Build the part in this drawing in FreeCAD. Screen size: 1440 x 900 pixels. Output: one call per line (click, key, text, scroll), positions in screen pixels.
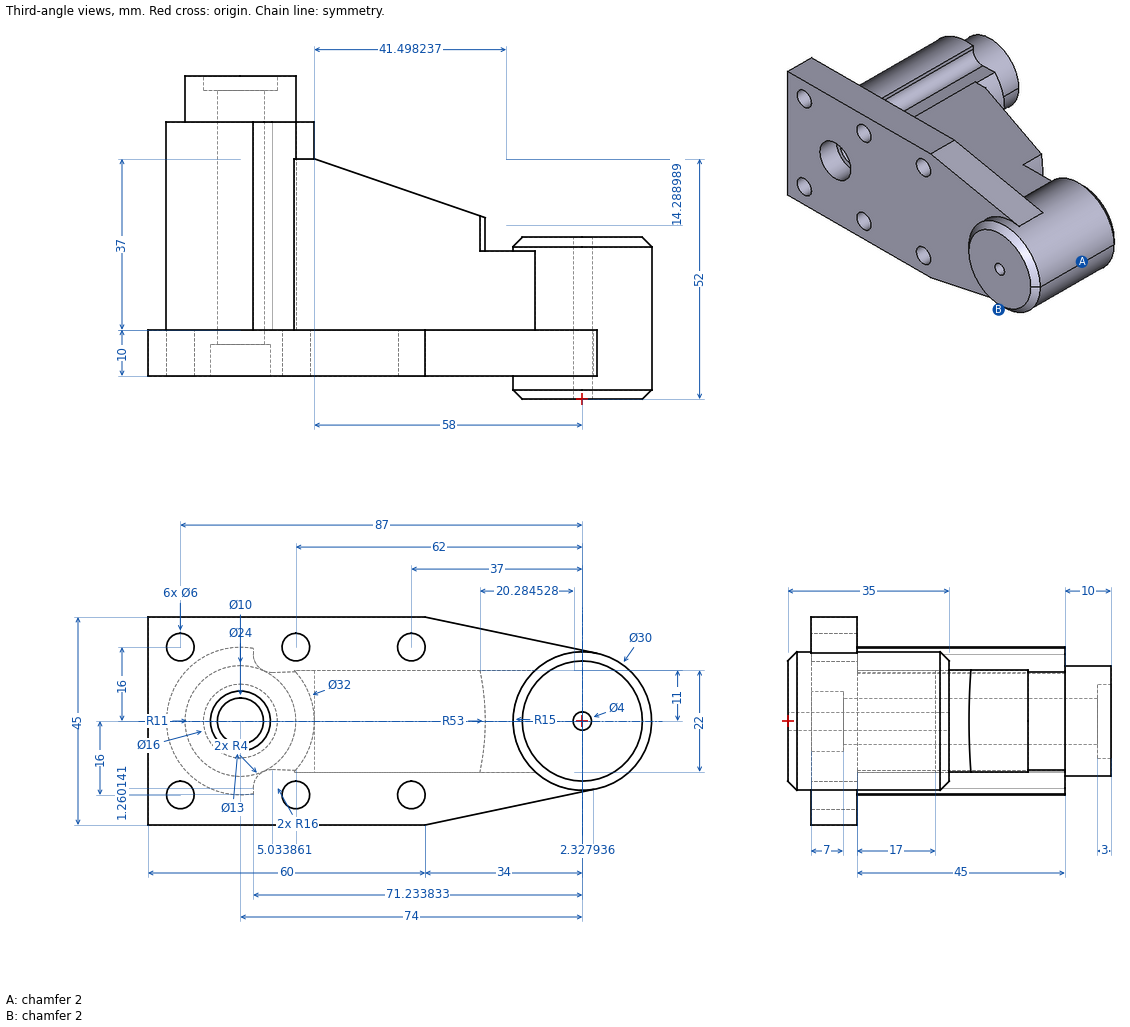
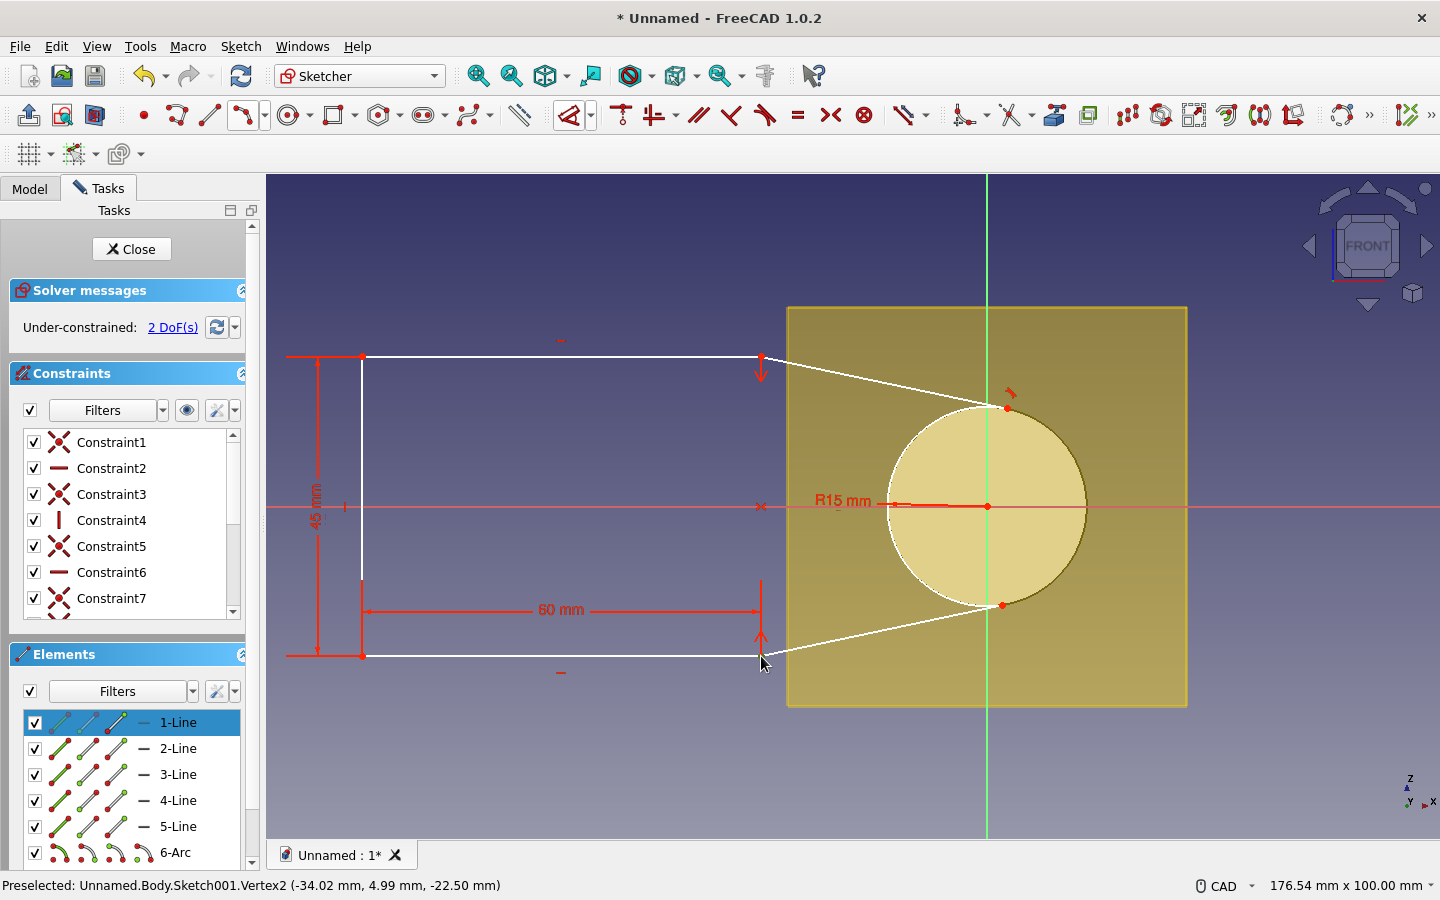
click(590, 116)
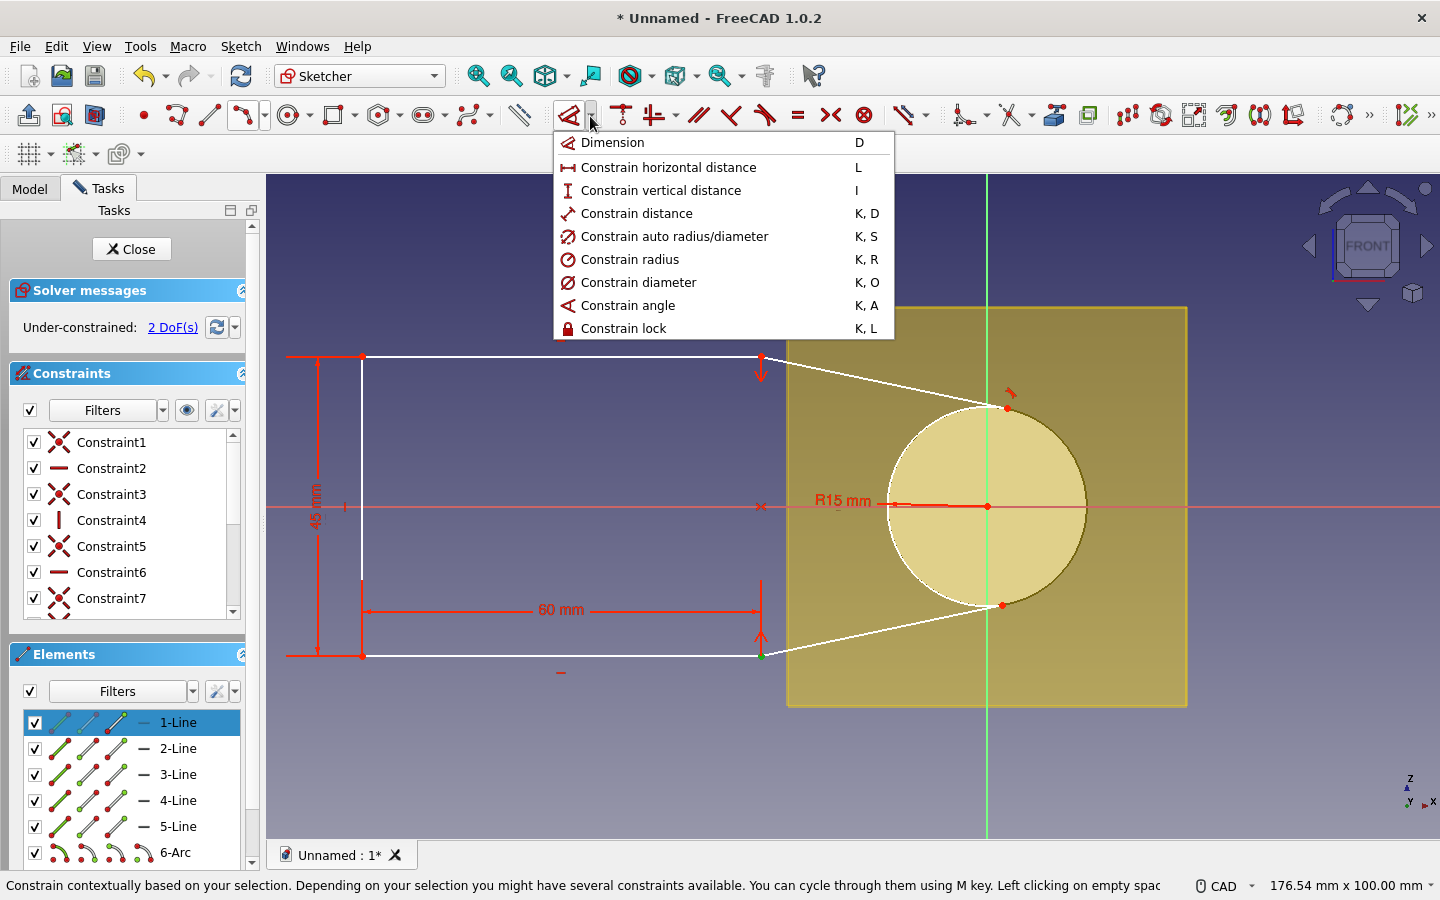
click(724, 168)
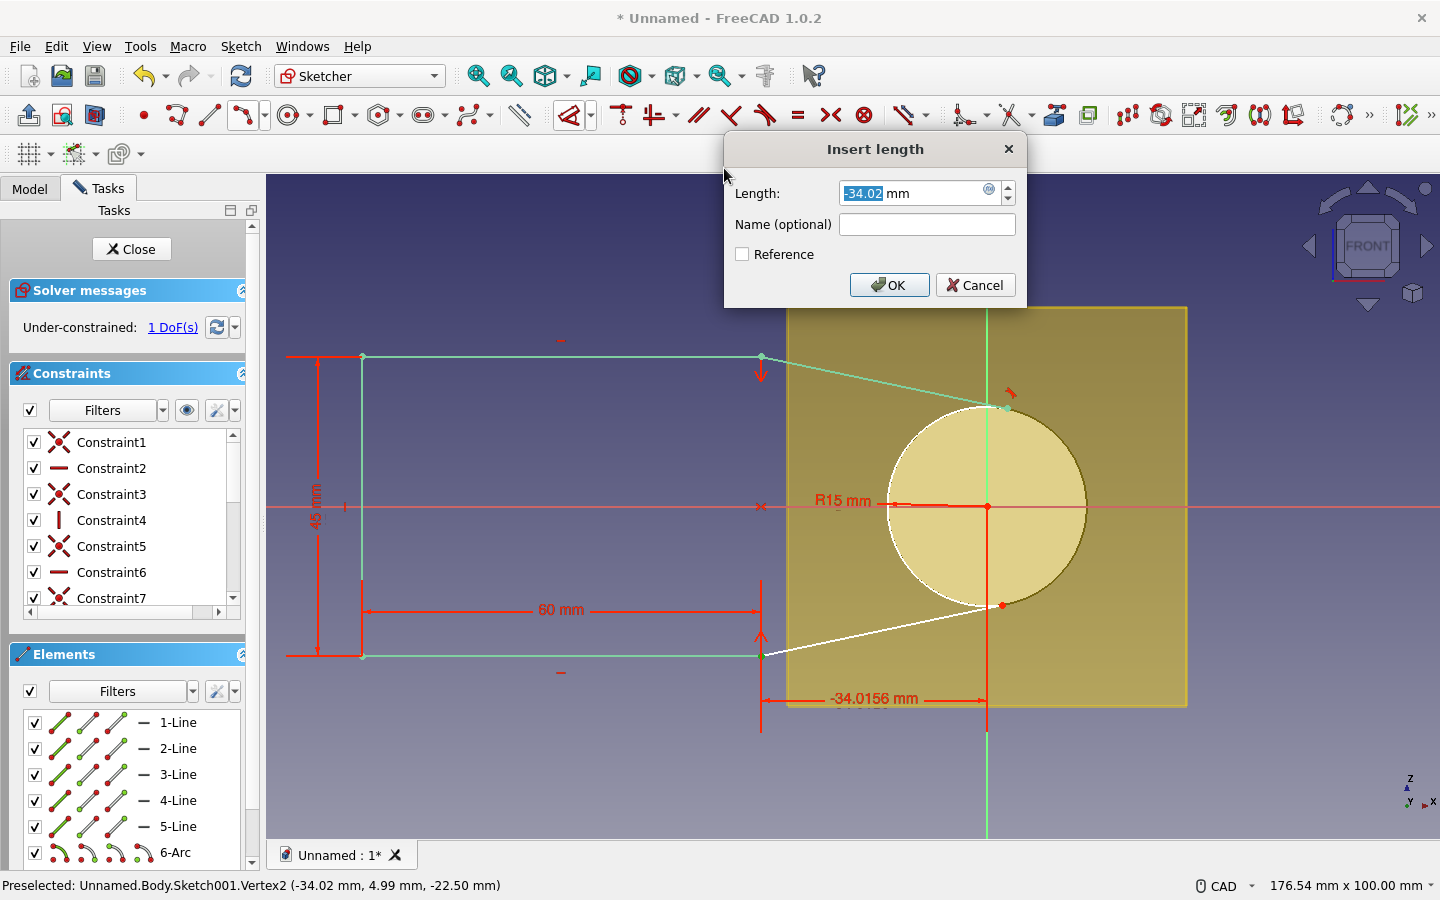
text(-34)
key(Return)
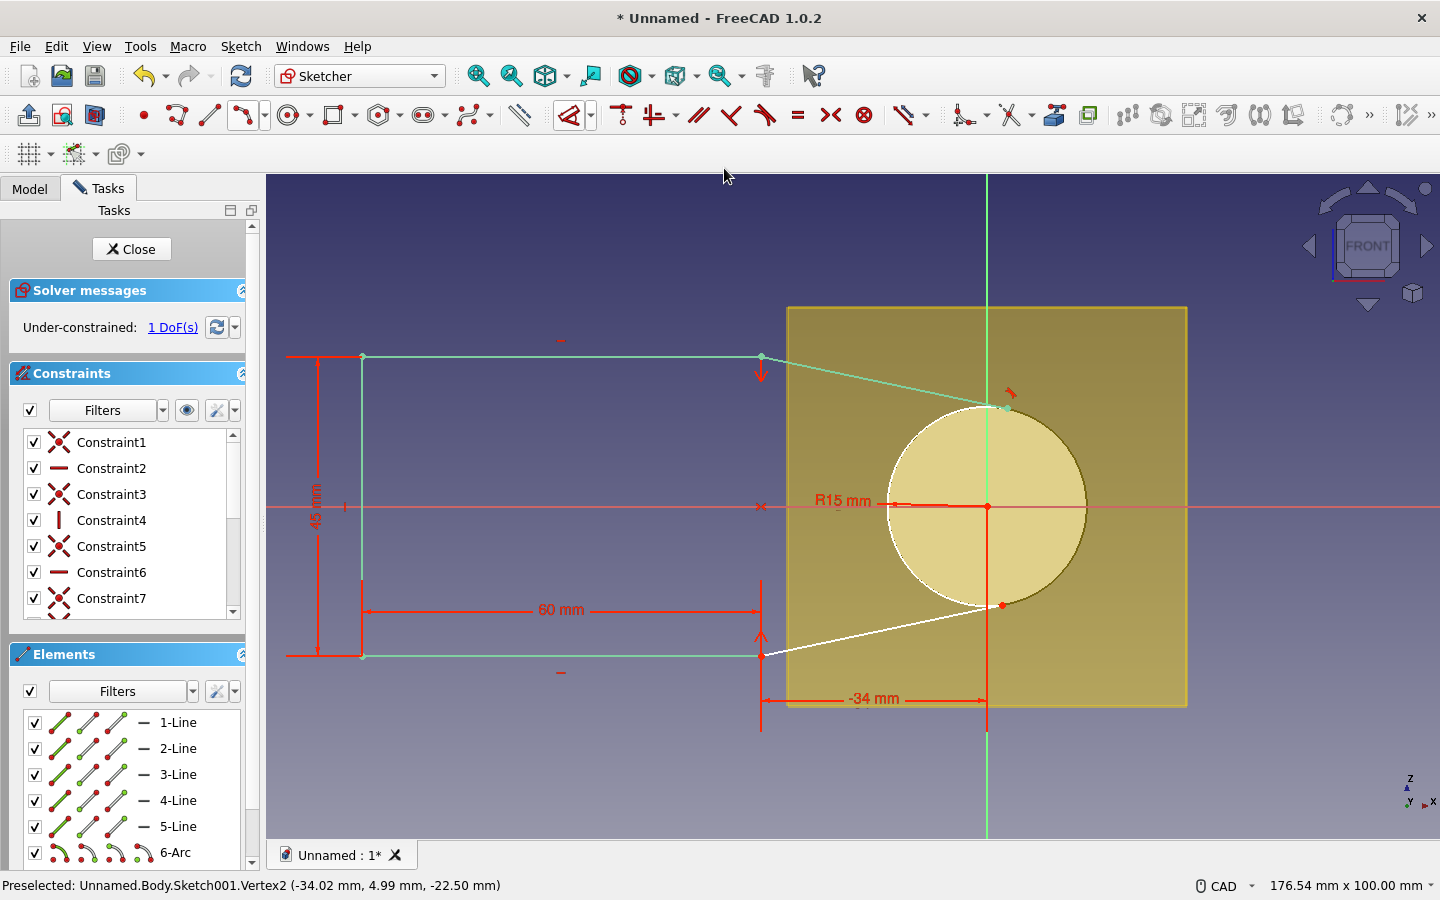
scroll(1003, 605, up, 5)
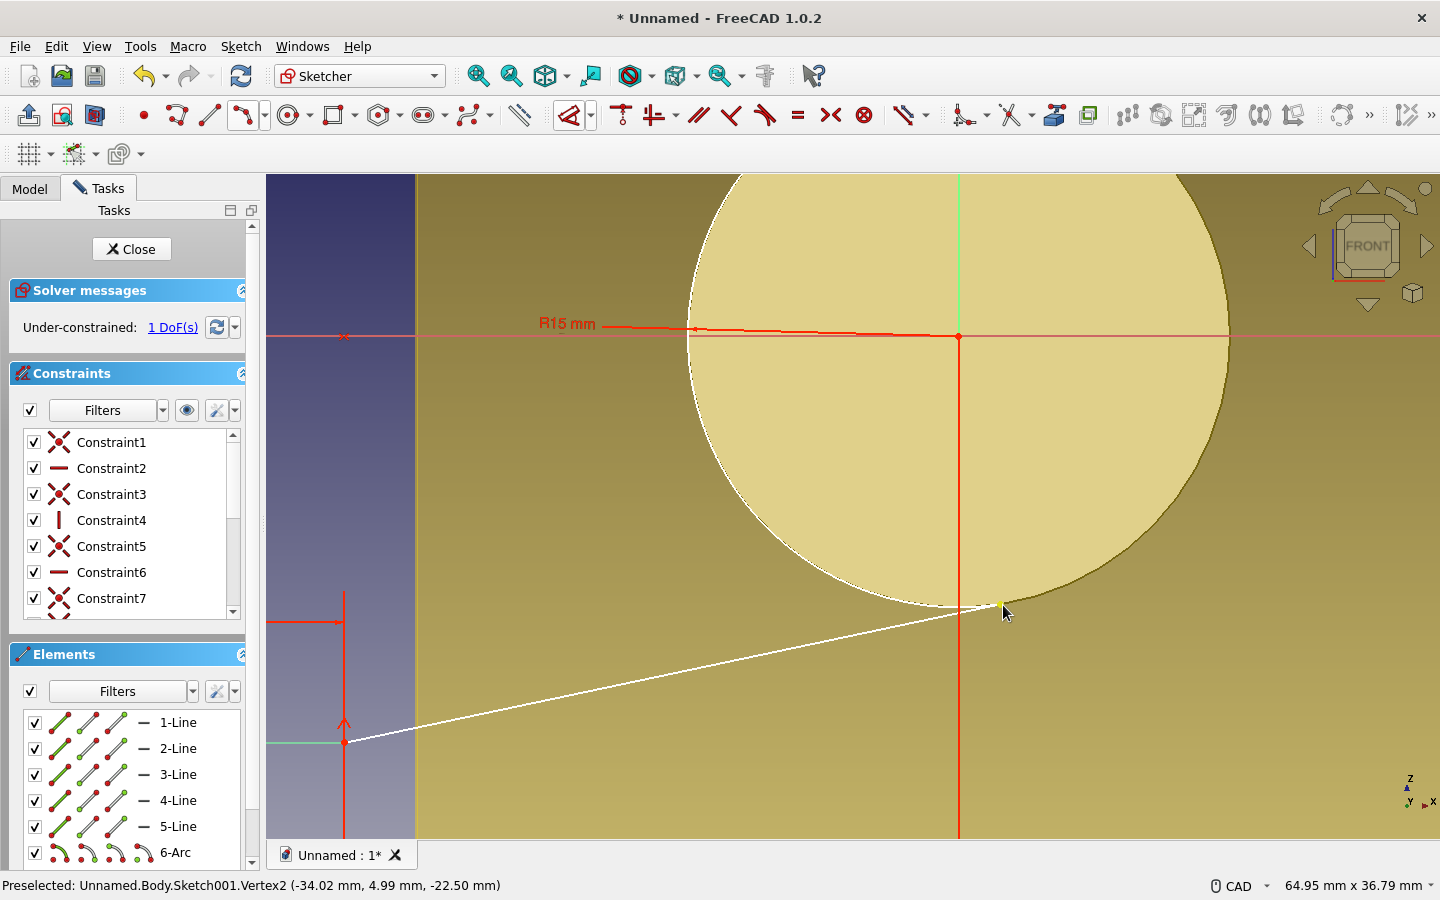
click(1001, 604)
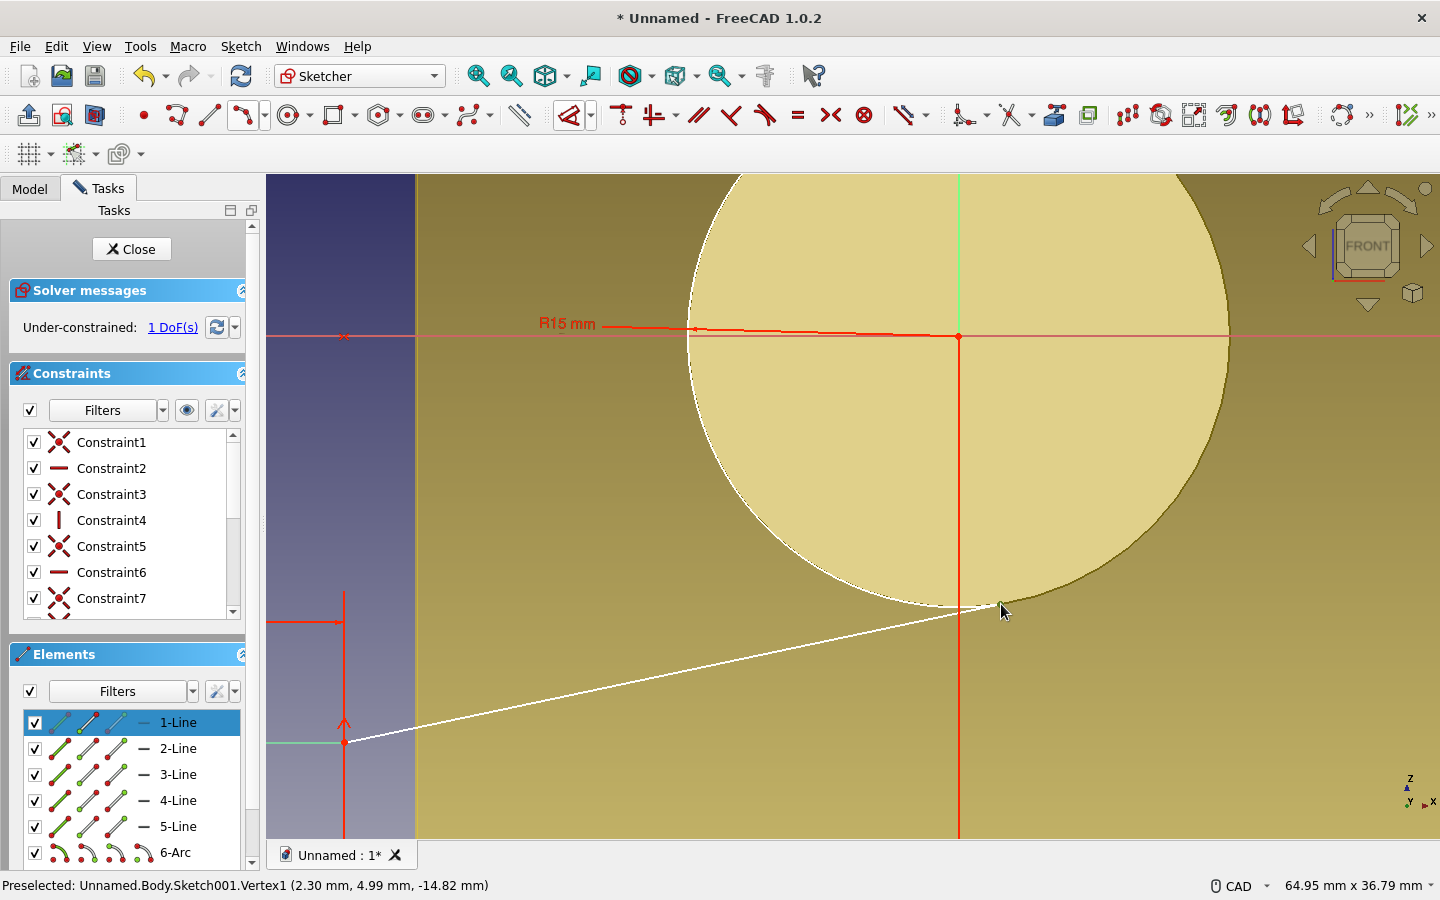
key(l)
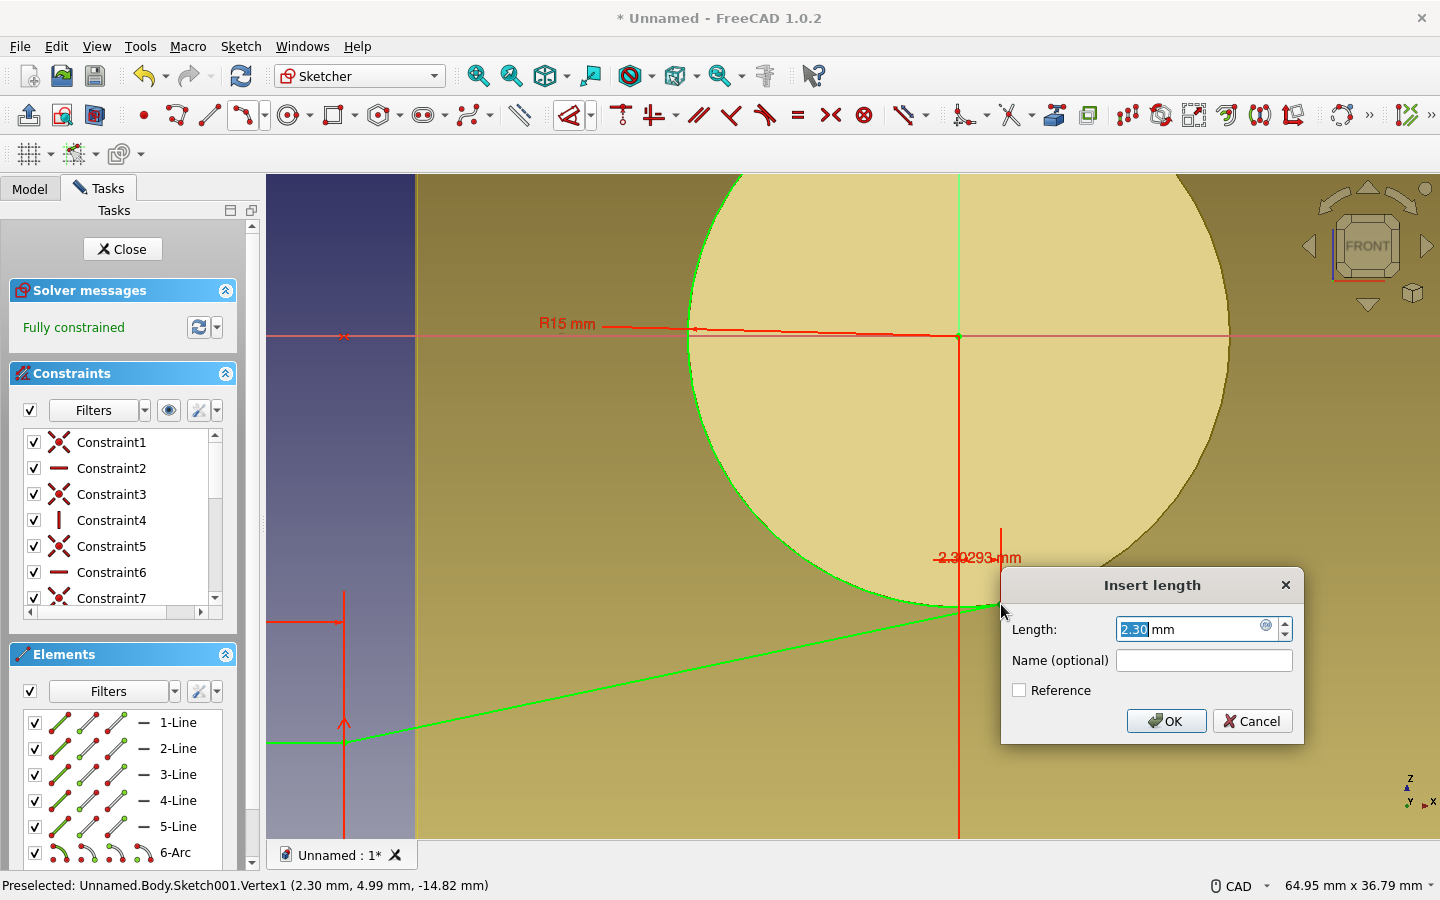
text(2.327936)
key(Return)